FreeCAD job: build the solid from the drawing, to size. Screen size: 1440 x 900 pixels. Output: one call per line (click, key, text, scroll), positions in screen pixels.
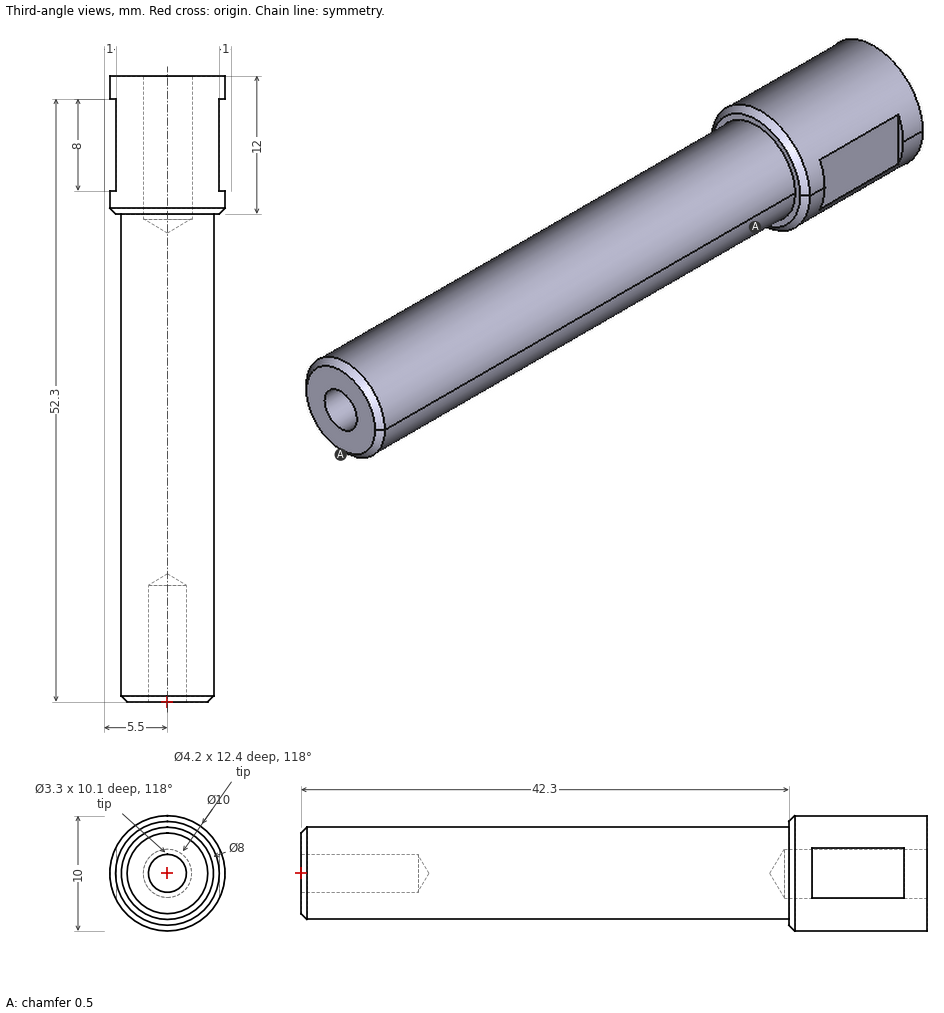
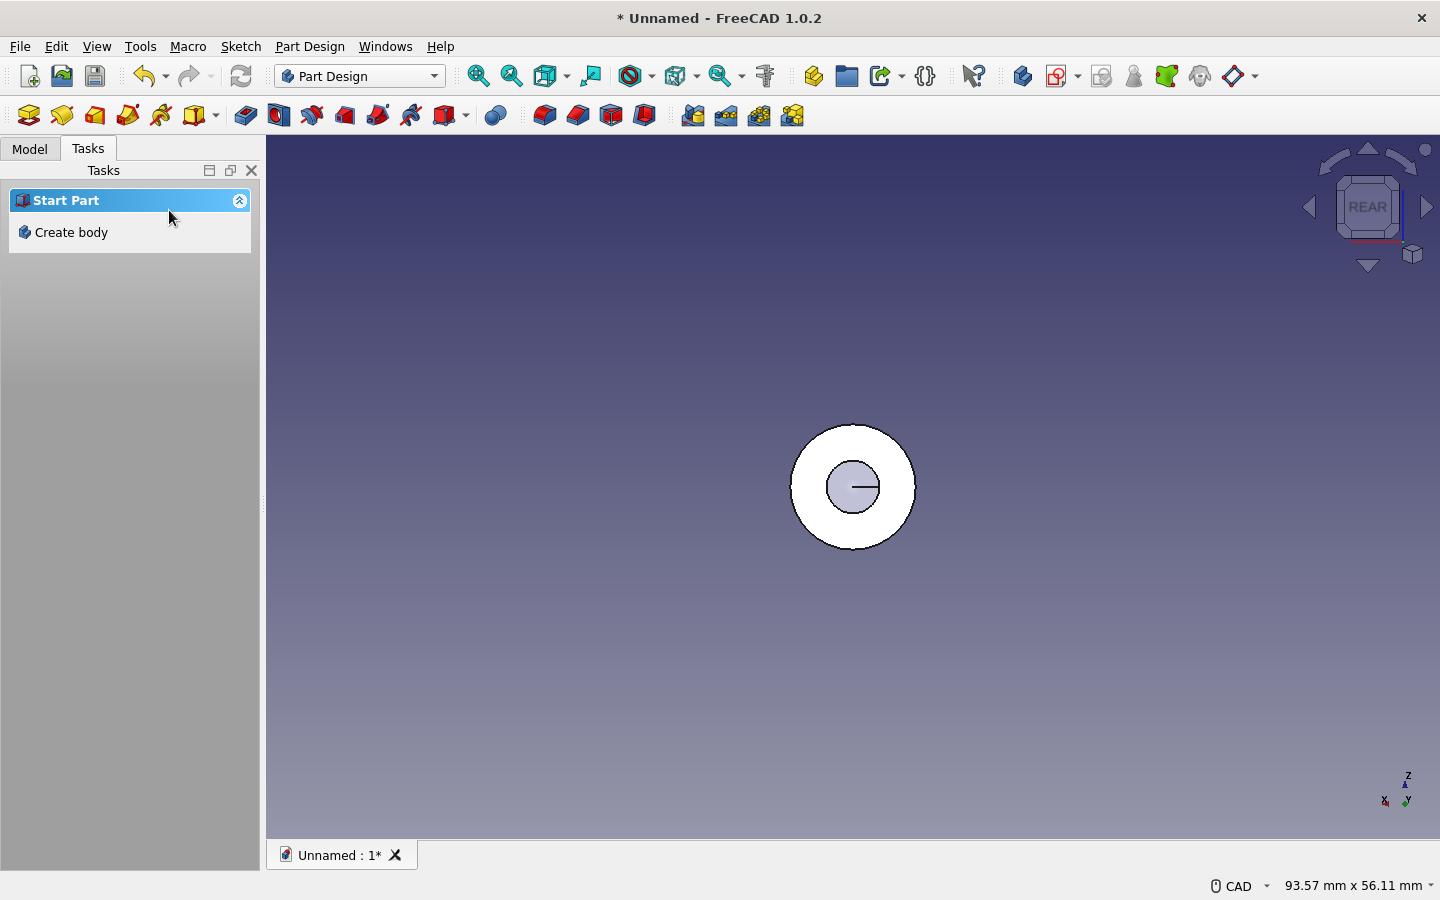
click(479, 76)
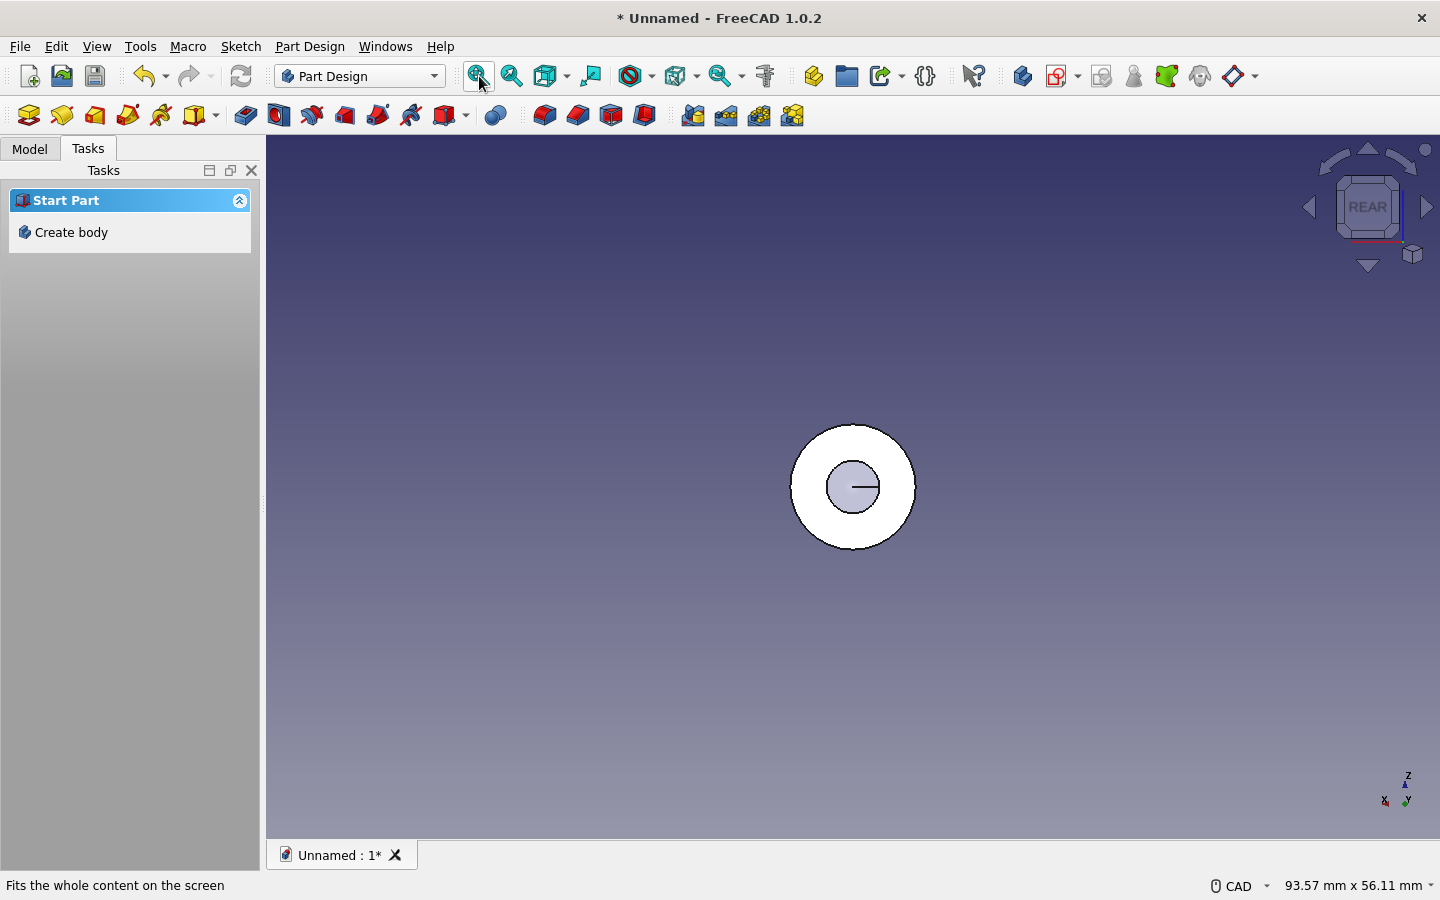
key(0)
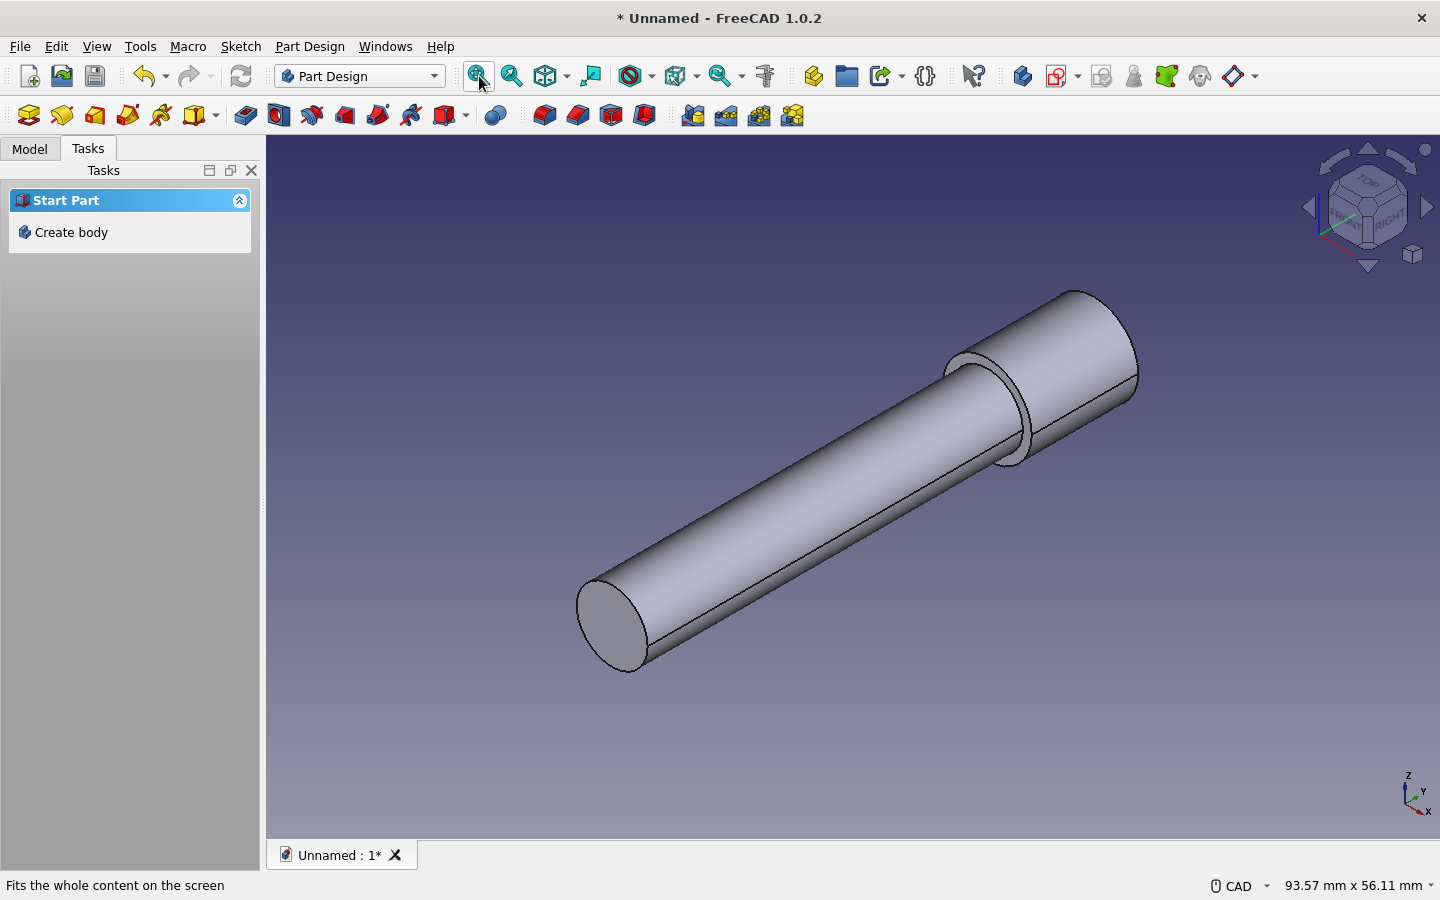
click(612, 625)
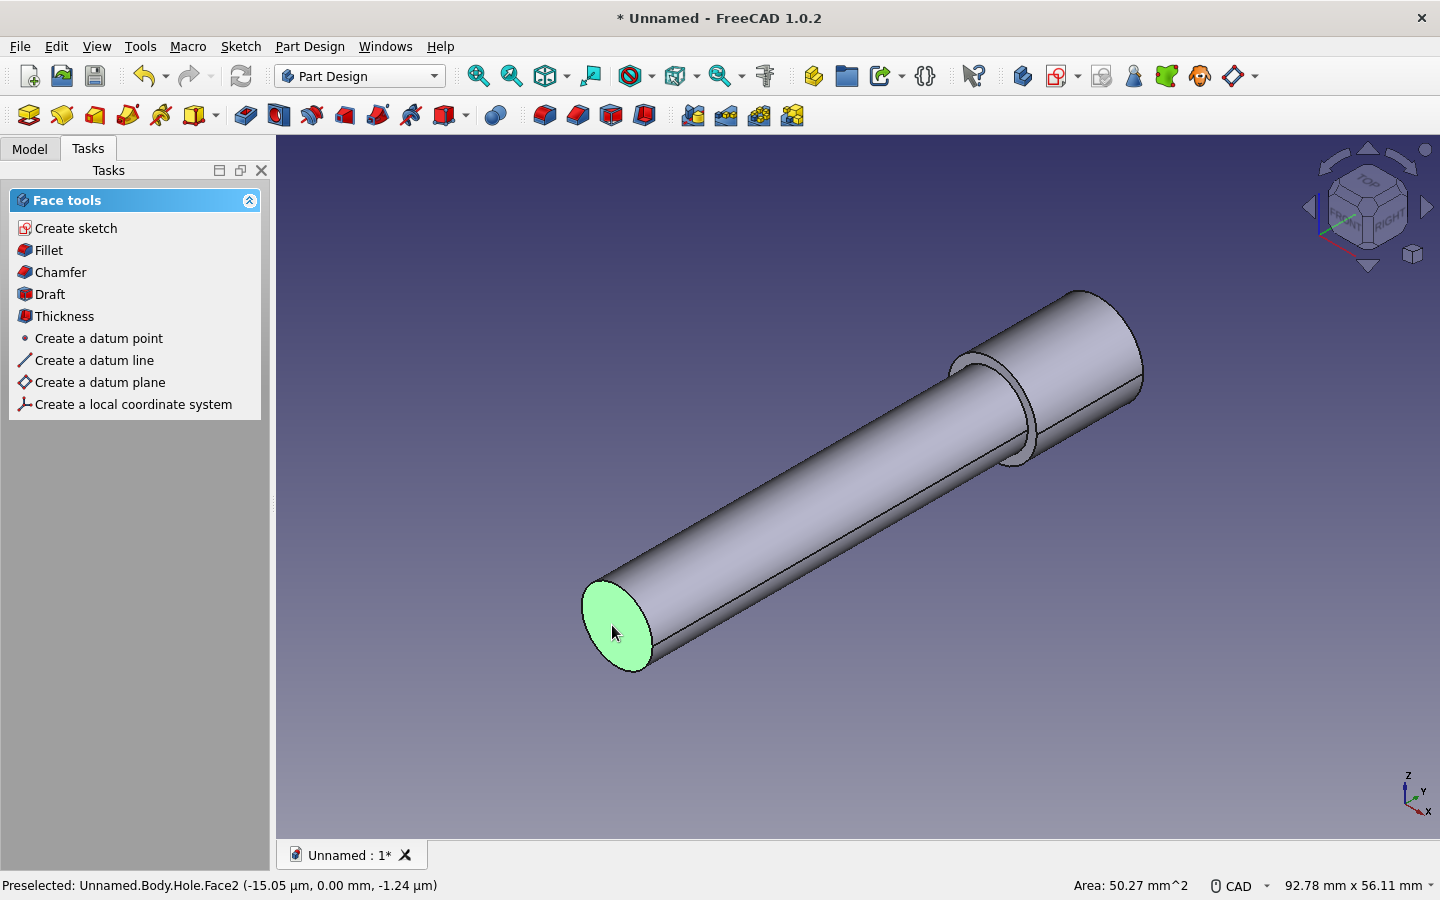
click(1056, 76)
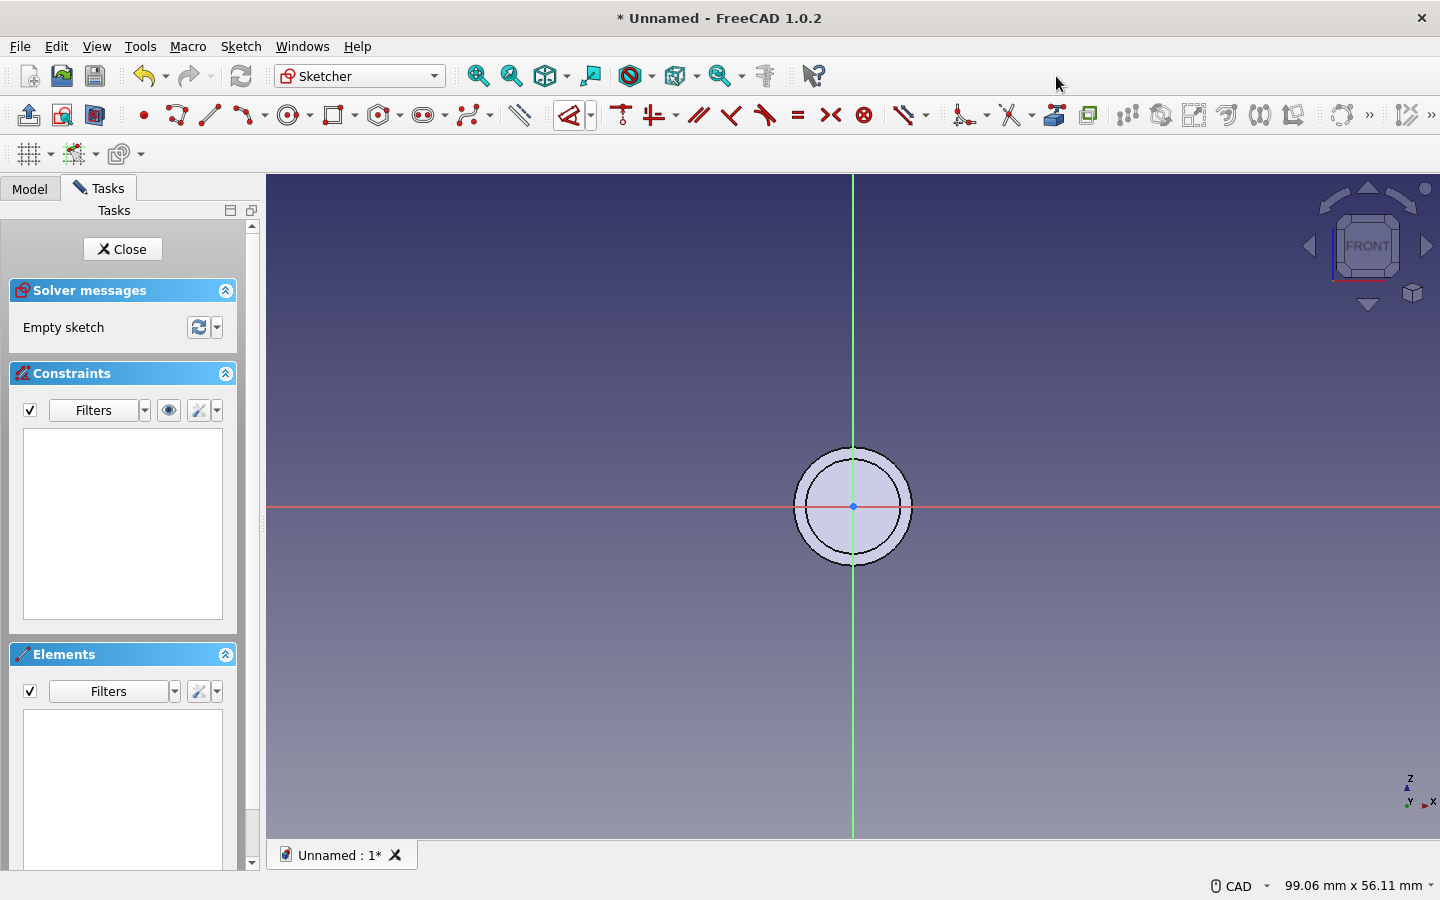
scroll(860, 507, up, 12)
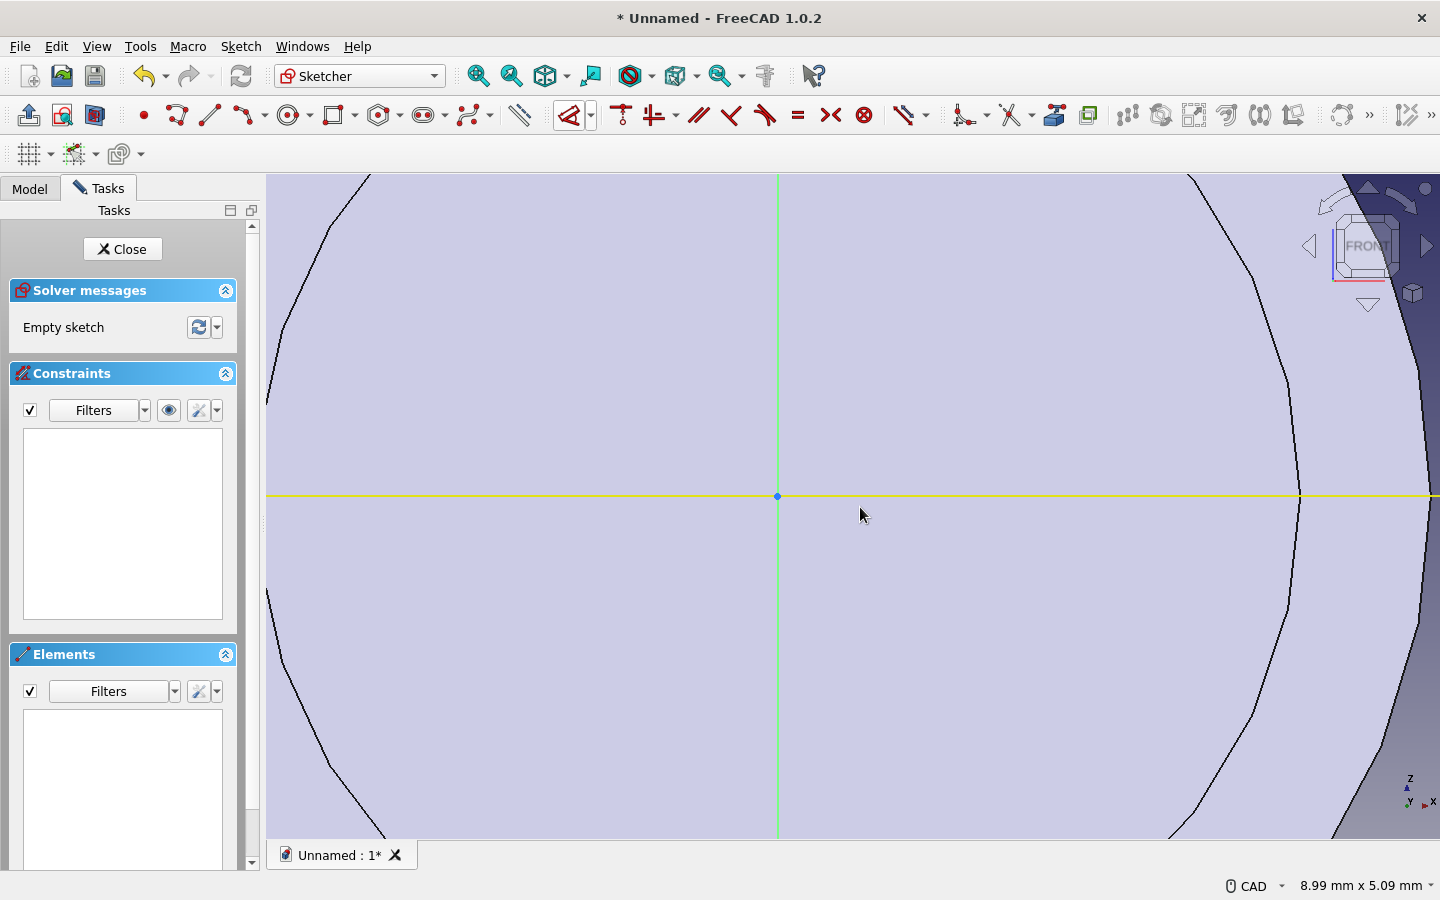
key(g)
key(c)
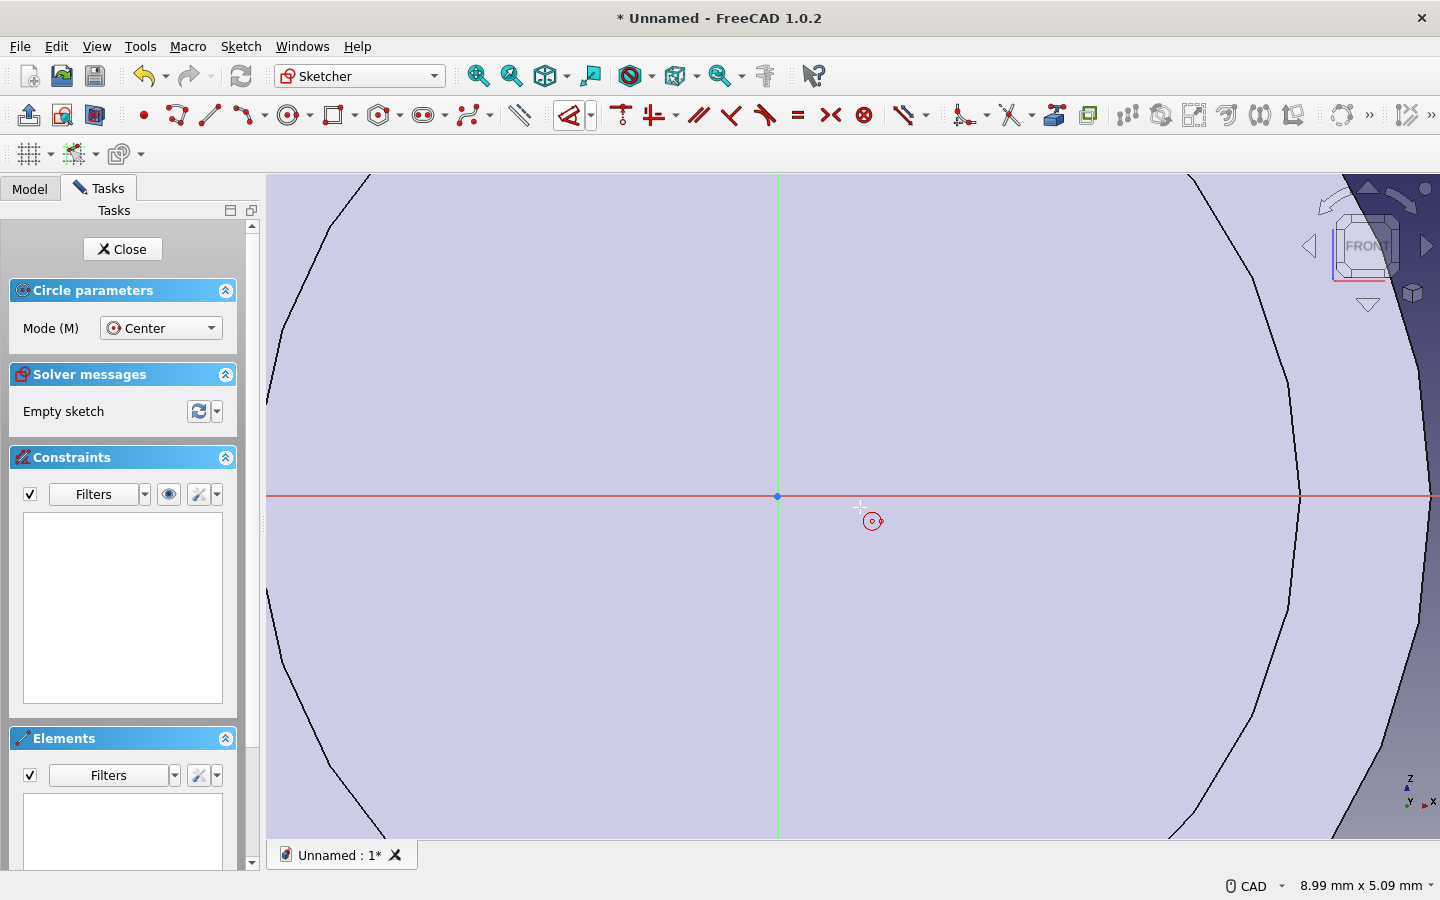
click(778, 496)
move(930, 344)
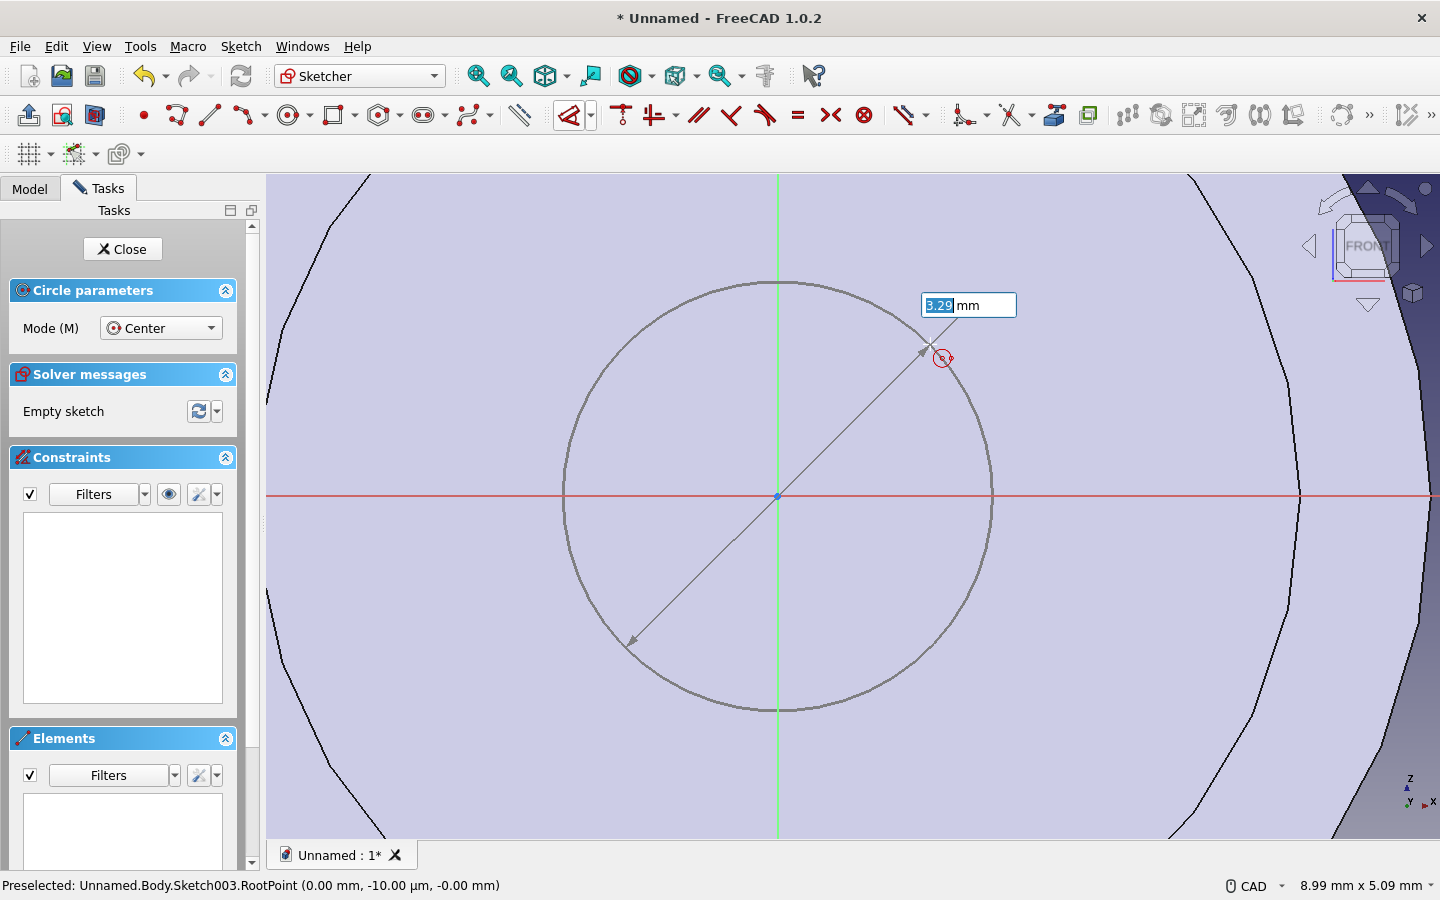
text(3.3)
key(Return)
key(Escape)